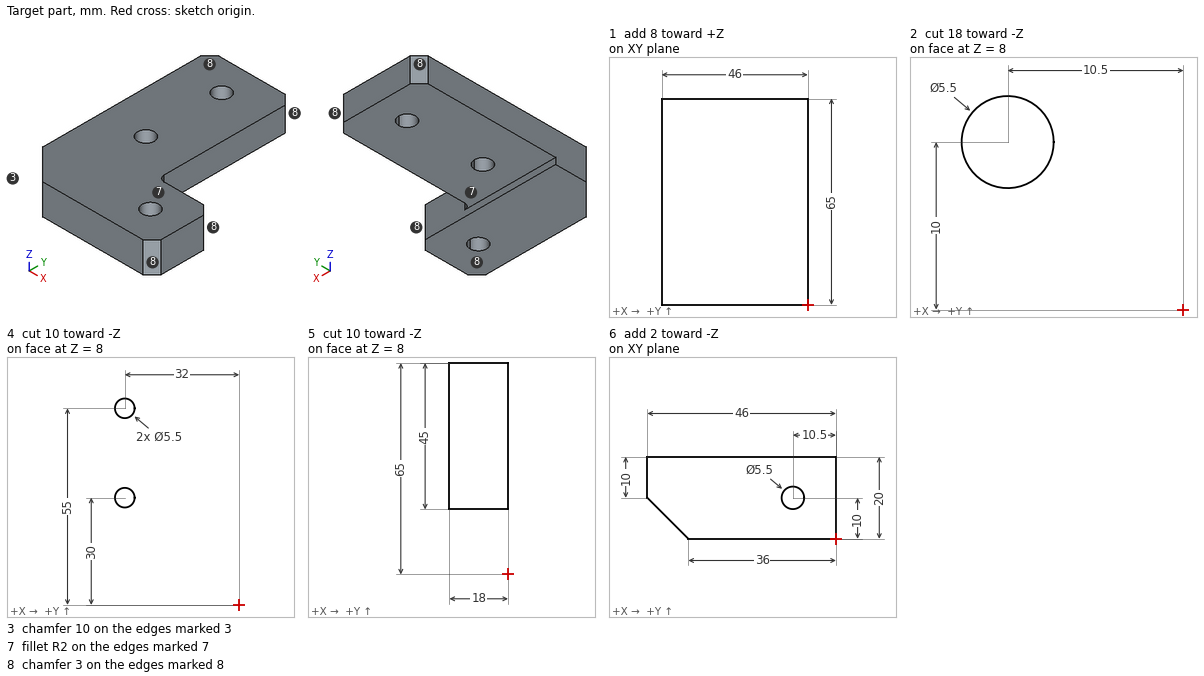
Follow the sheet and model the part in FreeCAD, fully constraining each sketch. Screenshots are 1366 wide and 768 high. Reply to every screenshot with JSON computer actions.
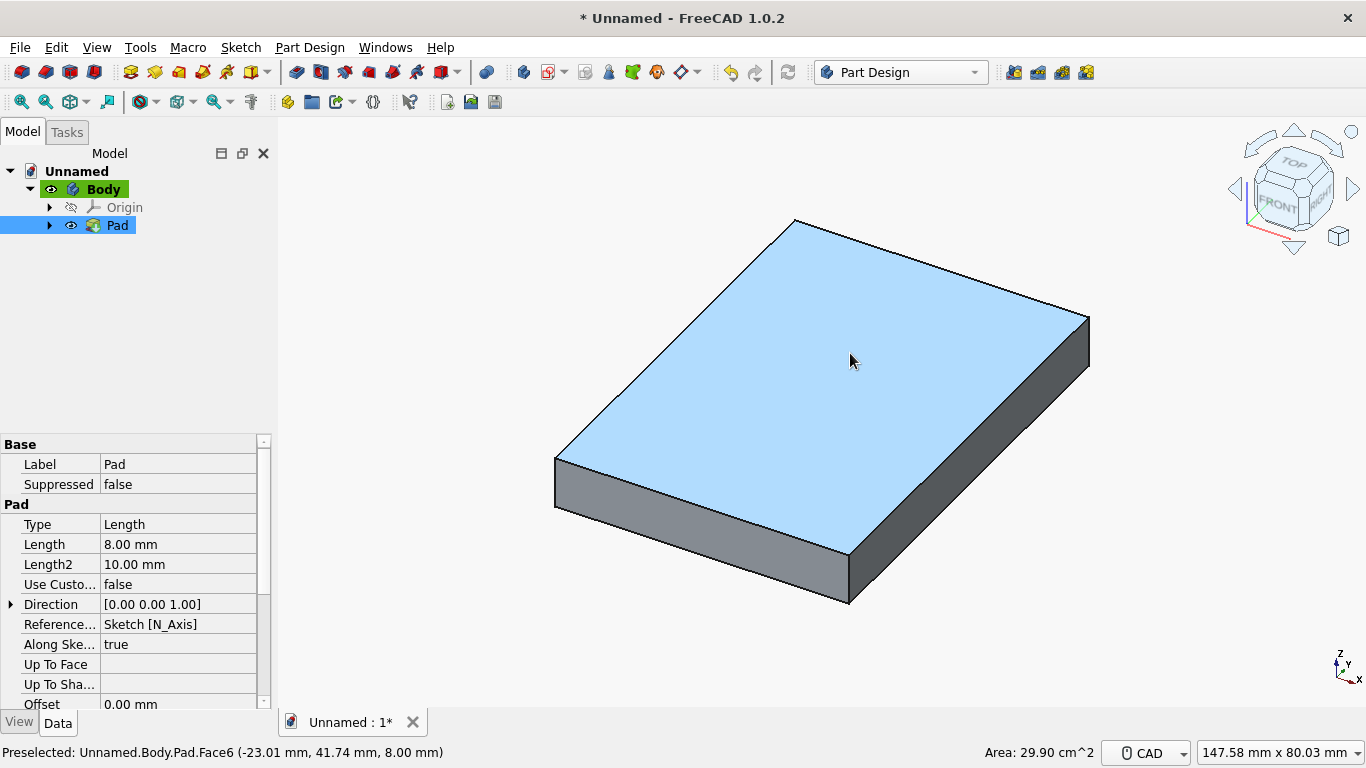
{"action": "left_click", "coordinate": [548, 72]}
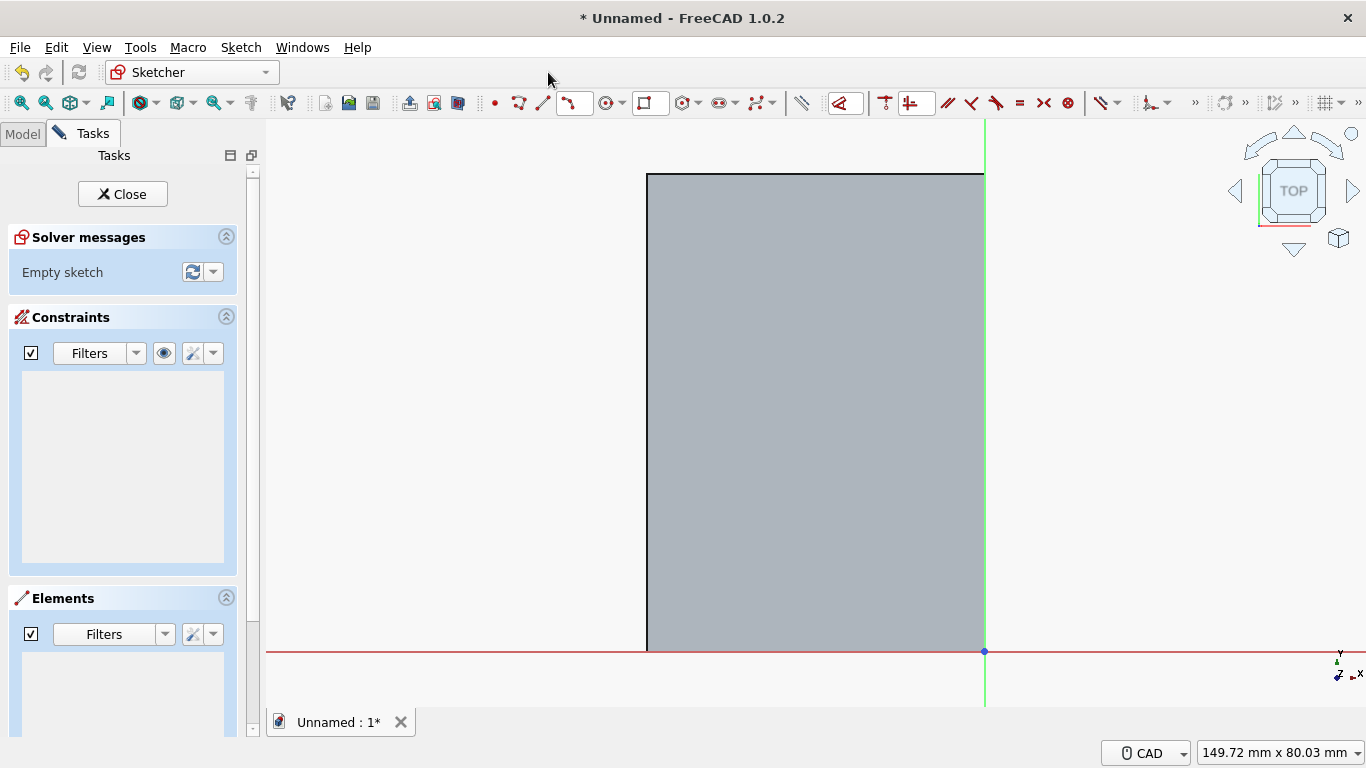
{"action": "scroll", "coordinate": [998, 668], "scroll_direction": "up", "scroll_amount": 7}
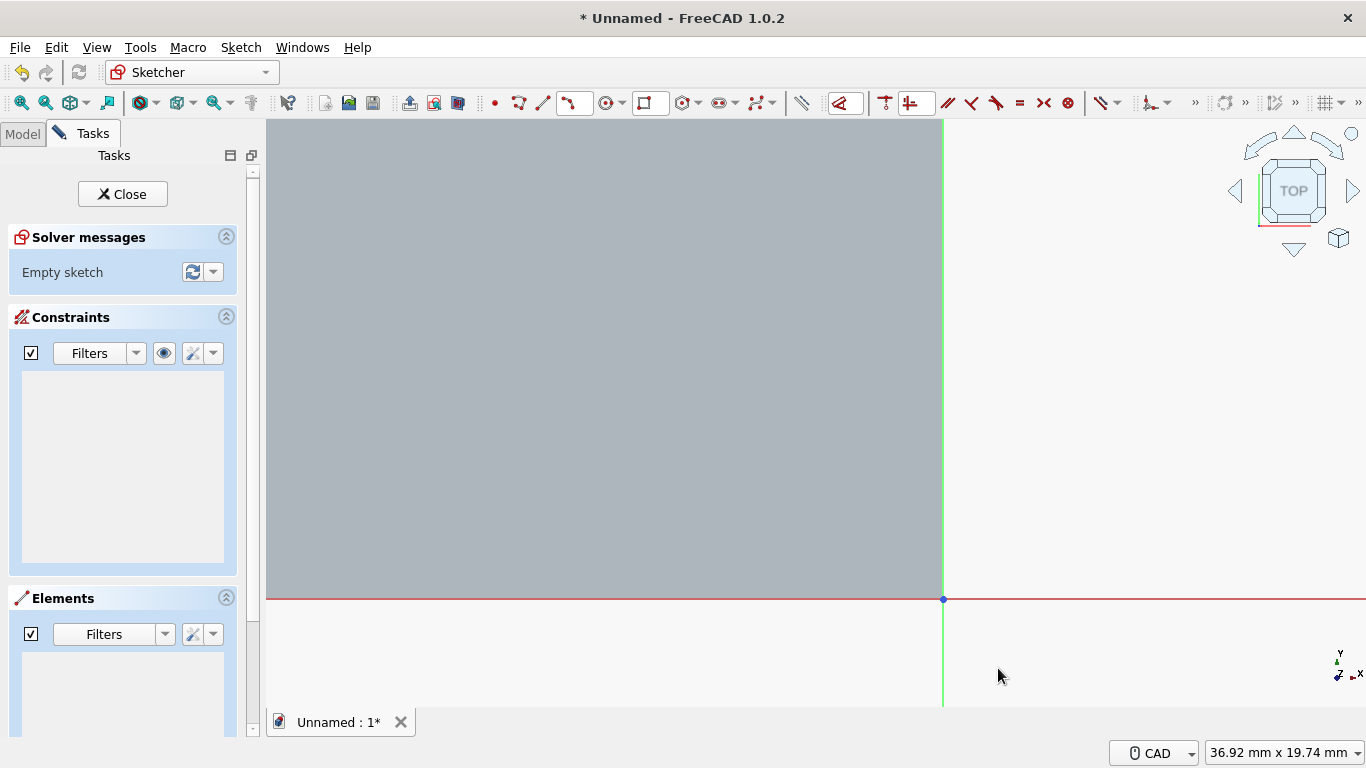
{"action": "left_click", "coordinate": [606, 104]}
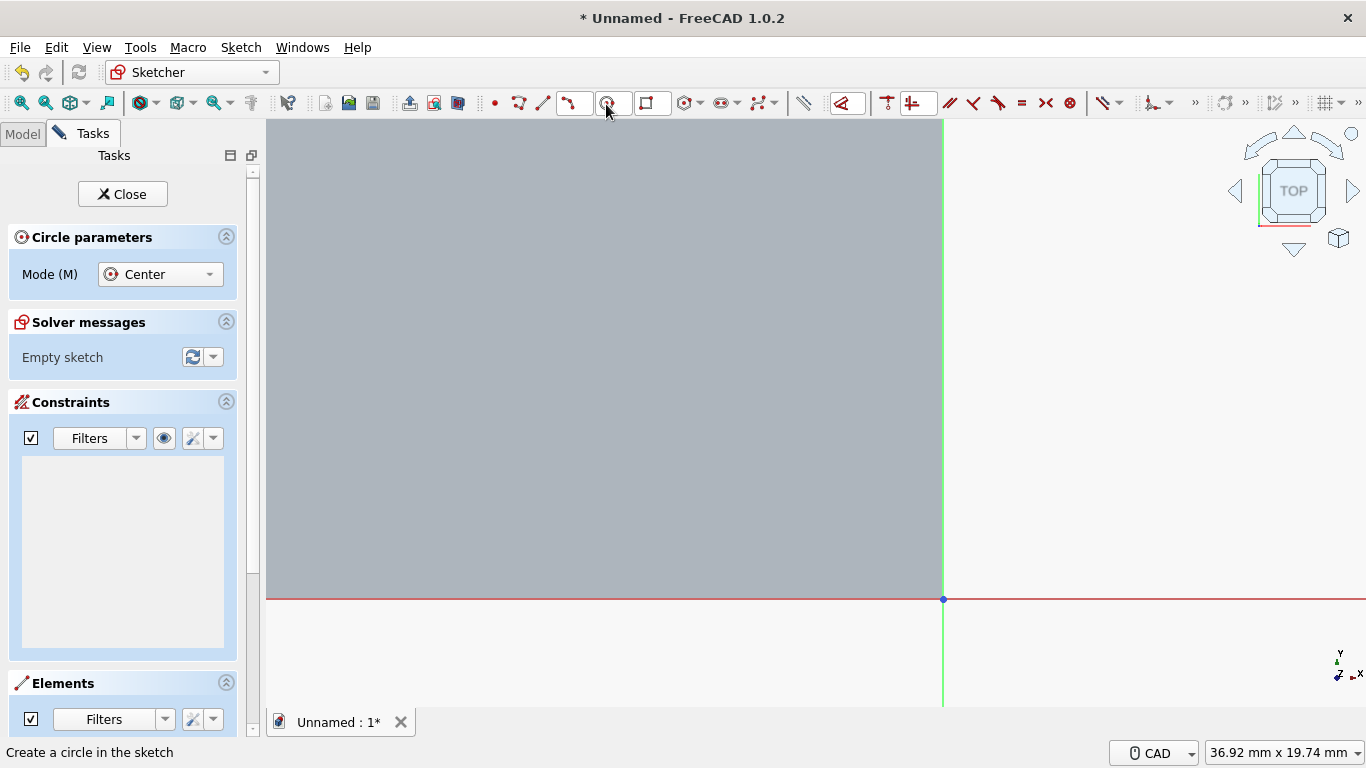
{"action": "left_click", "coordinate": [630, 301]}
{"action": "left_click", "coordinate": [688, 243]}
{"action": "key", "text": "Escape"}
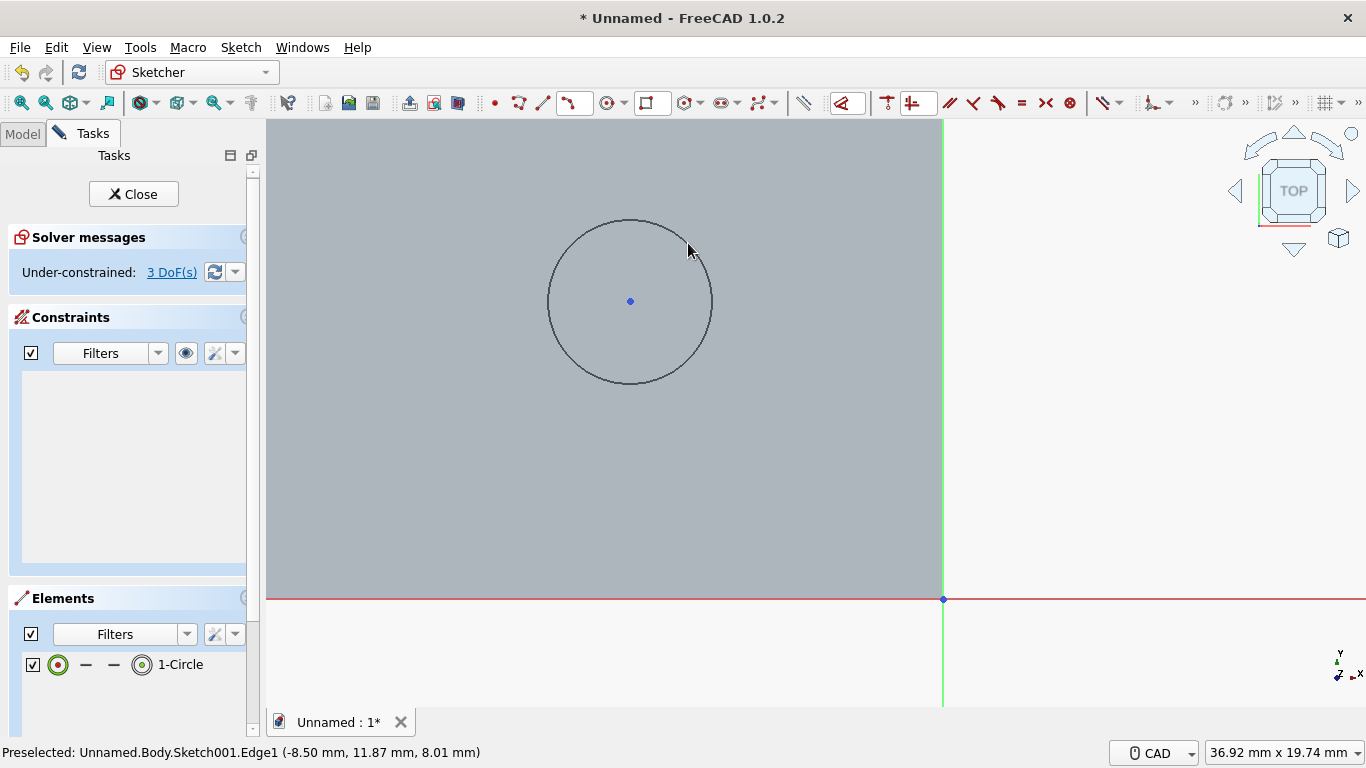
{"action": "left_click", "coordinate": [688, 244]}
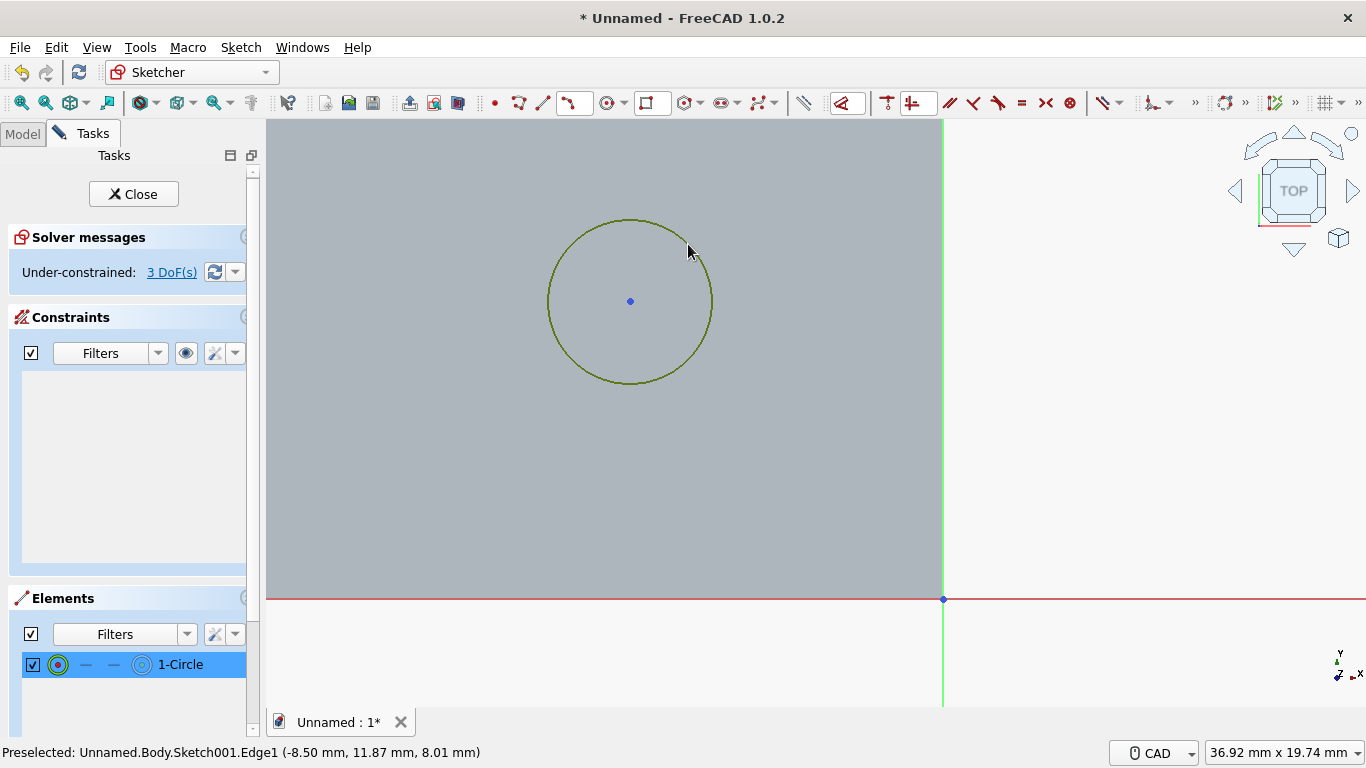
{"action": "left_click", "coordinate": [860, 104]}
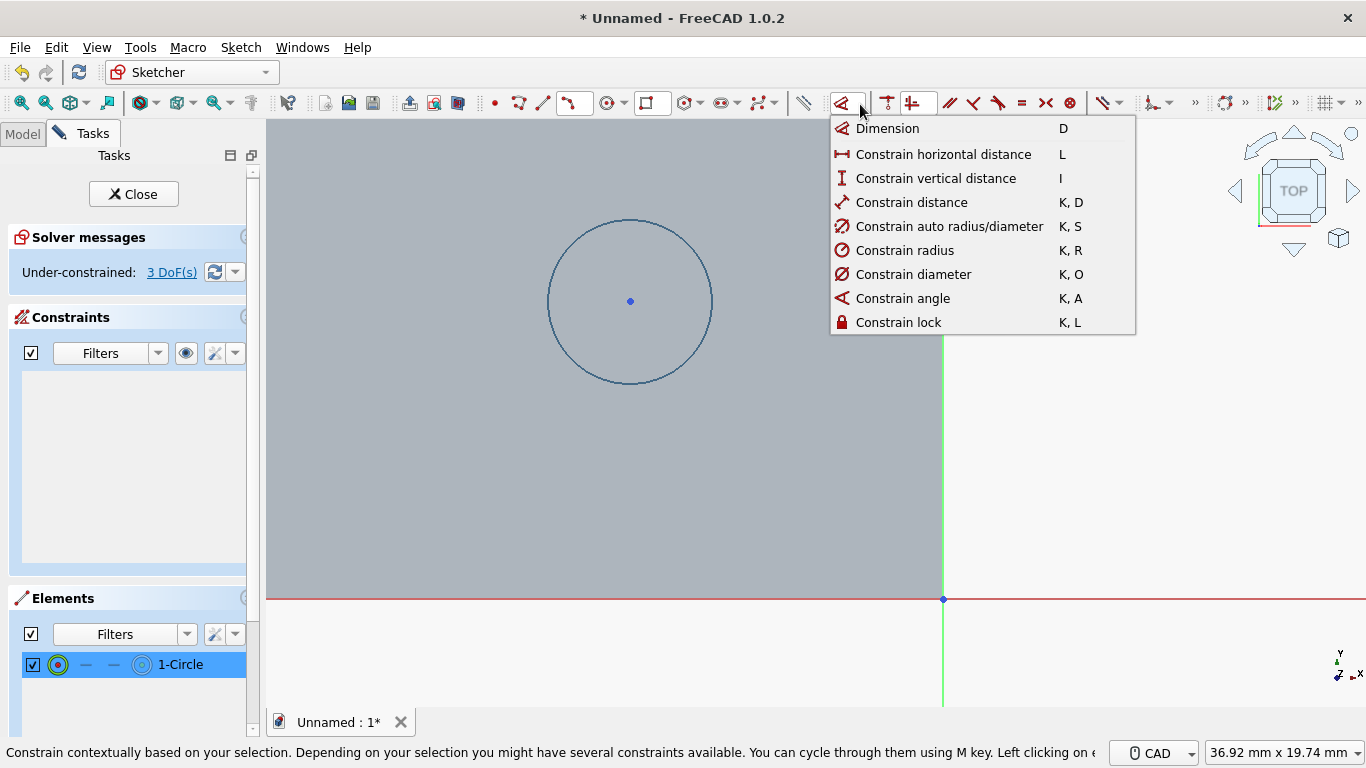
{"action": "left_click", "coordinate": [983, 274]}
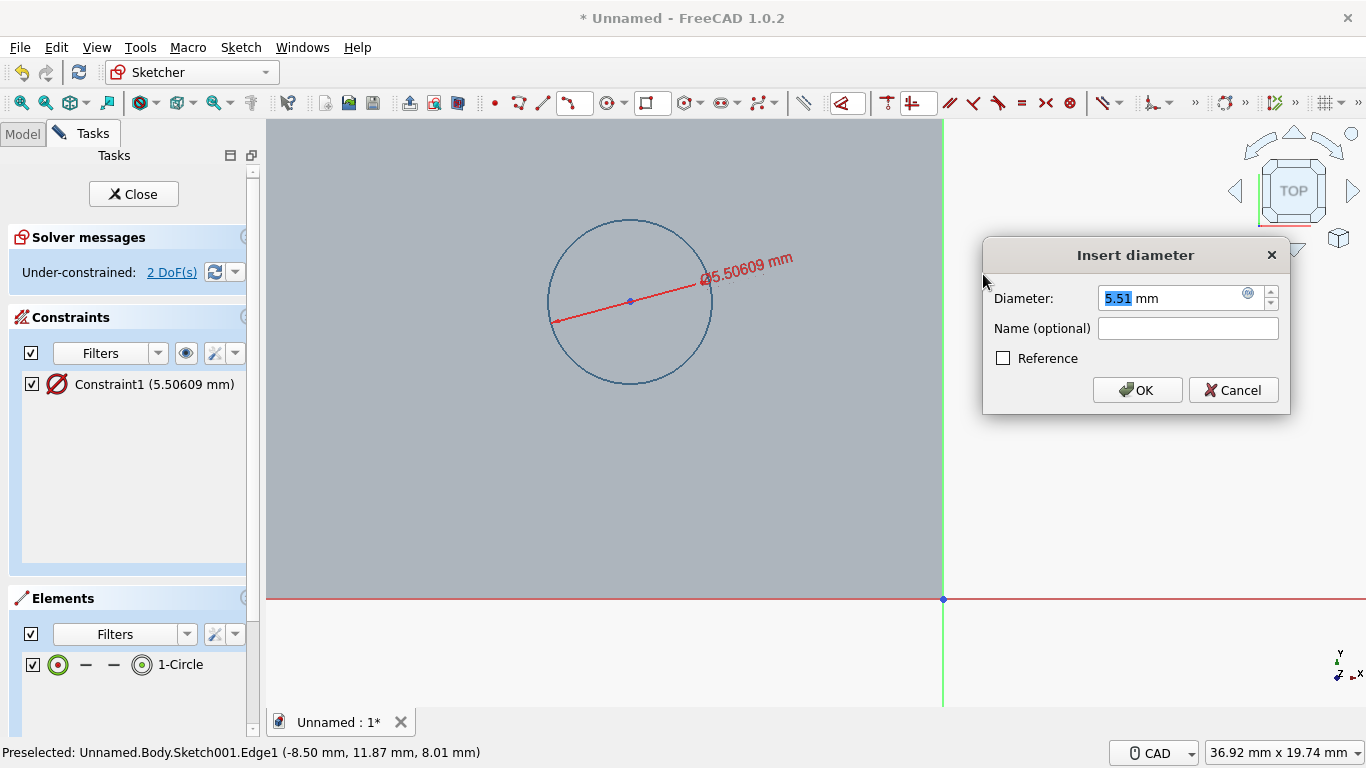
{"action": "type", "text": "5.5"}
{"action": "key", "text": "Return"}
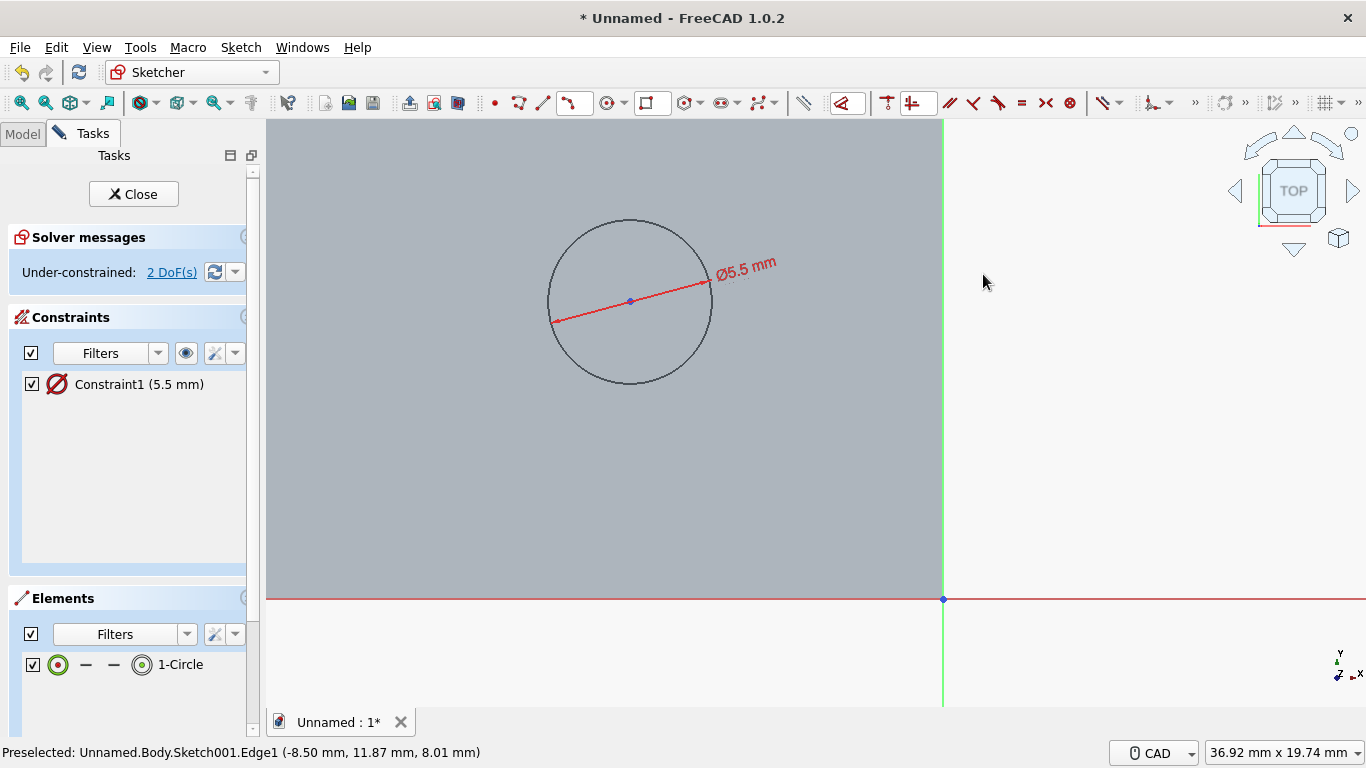
{"action": "left_click", "coordinate": [630, 302]}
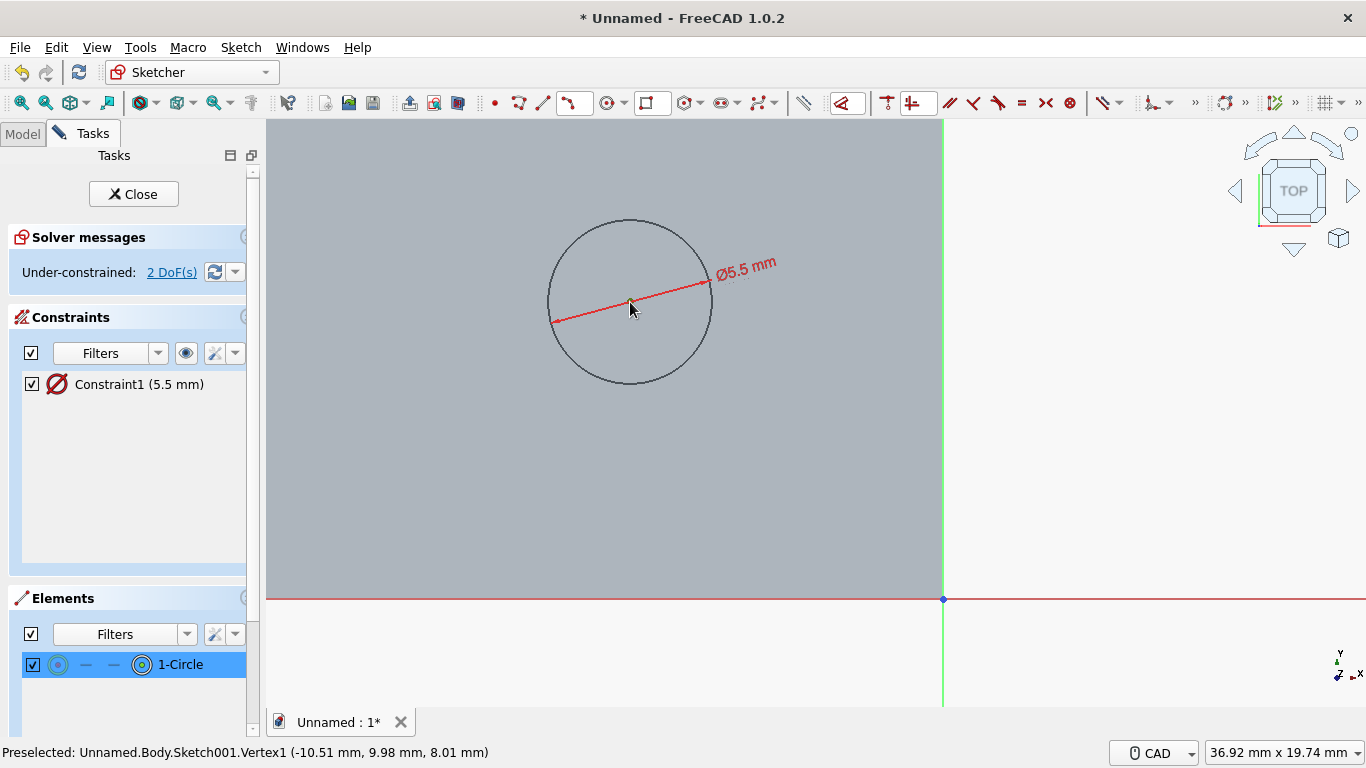
{"action": "left_click", "coordinate": [860, 104]}